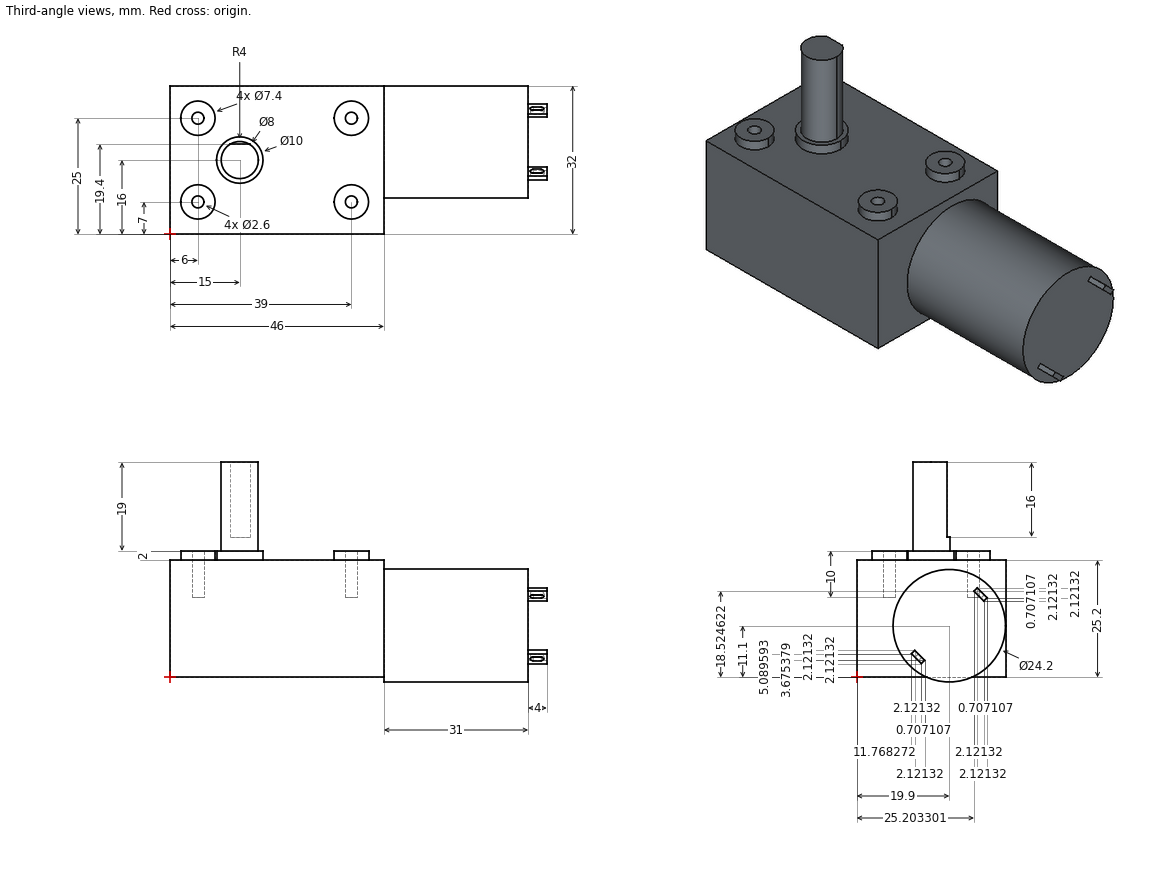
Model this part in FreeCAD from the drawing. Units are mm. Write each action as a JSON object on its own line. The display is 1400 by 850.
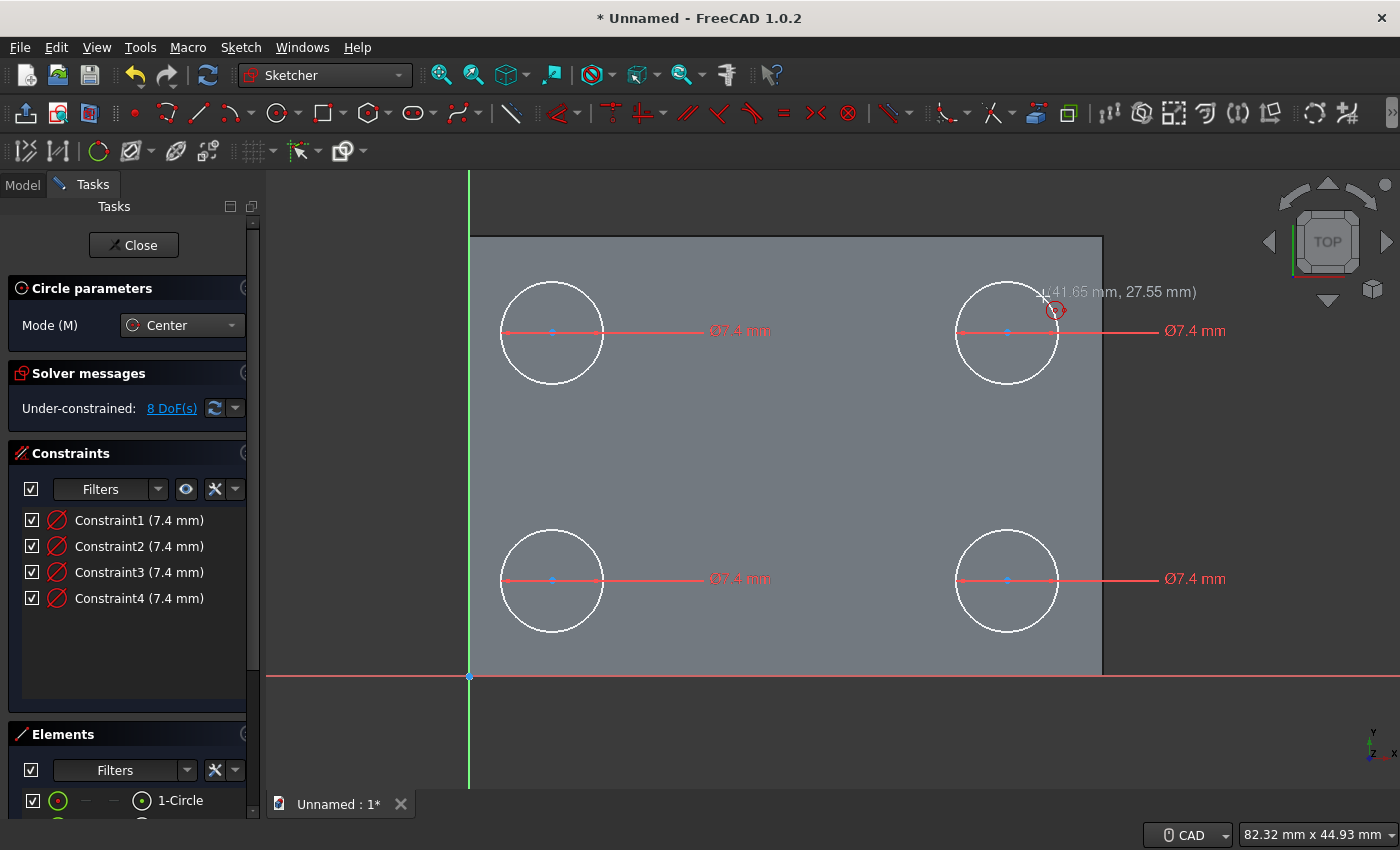
{"action": "left_click", "coordinate": [676, 456]}
{"action": "mouse_move", "coordinate": [725, 407]}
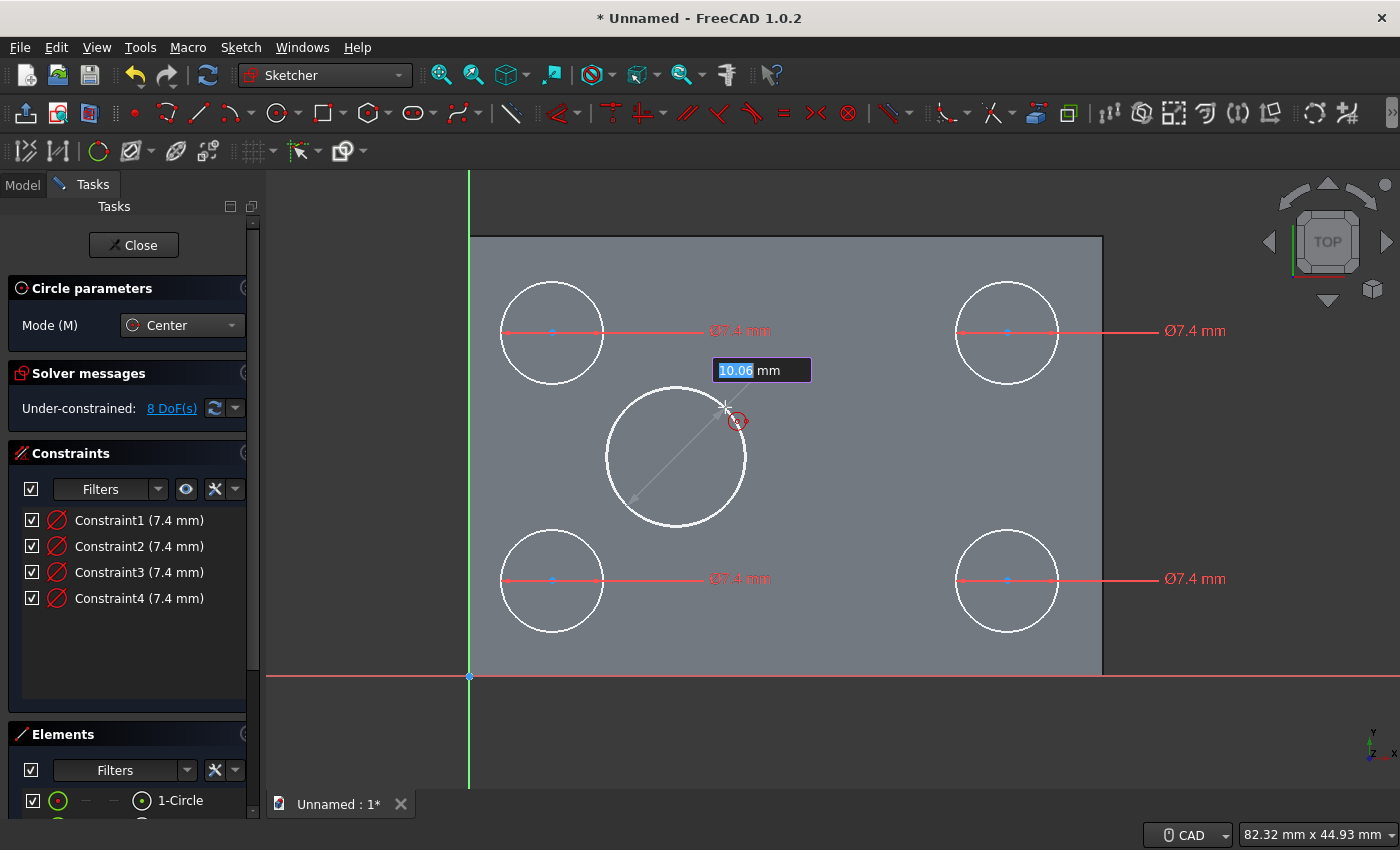
{"action": "type", "text": "10"}
{"action": "key", "text": "Return"}
{"action": "key", "text": "Escape"}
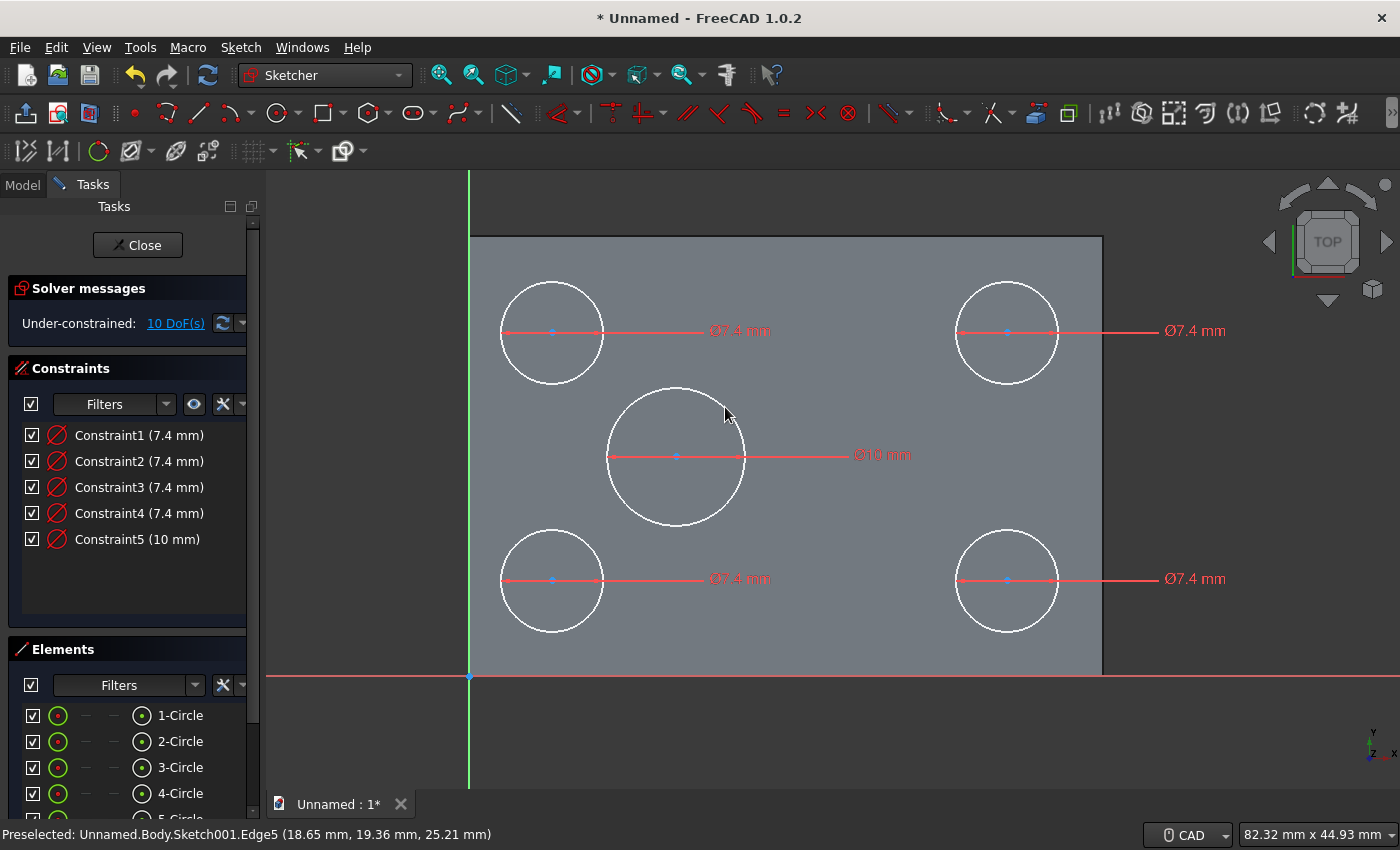
{"action": "left_click", "coordinate": [552, 333]}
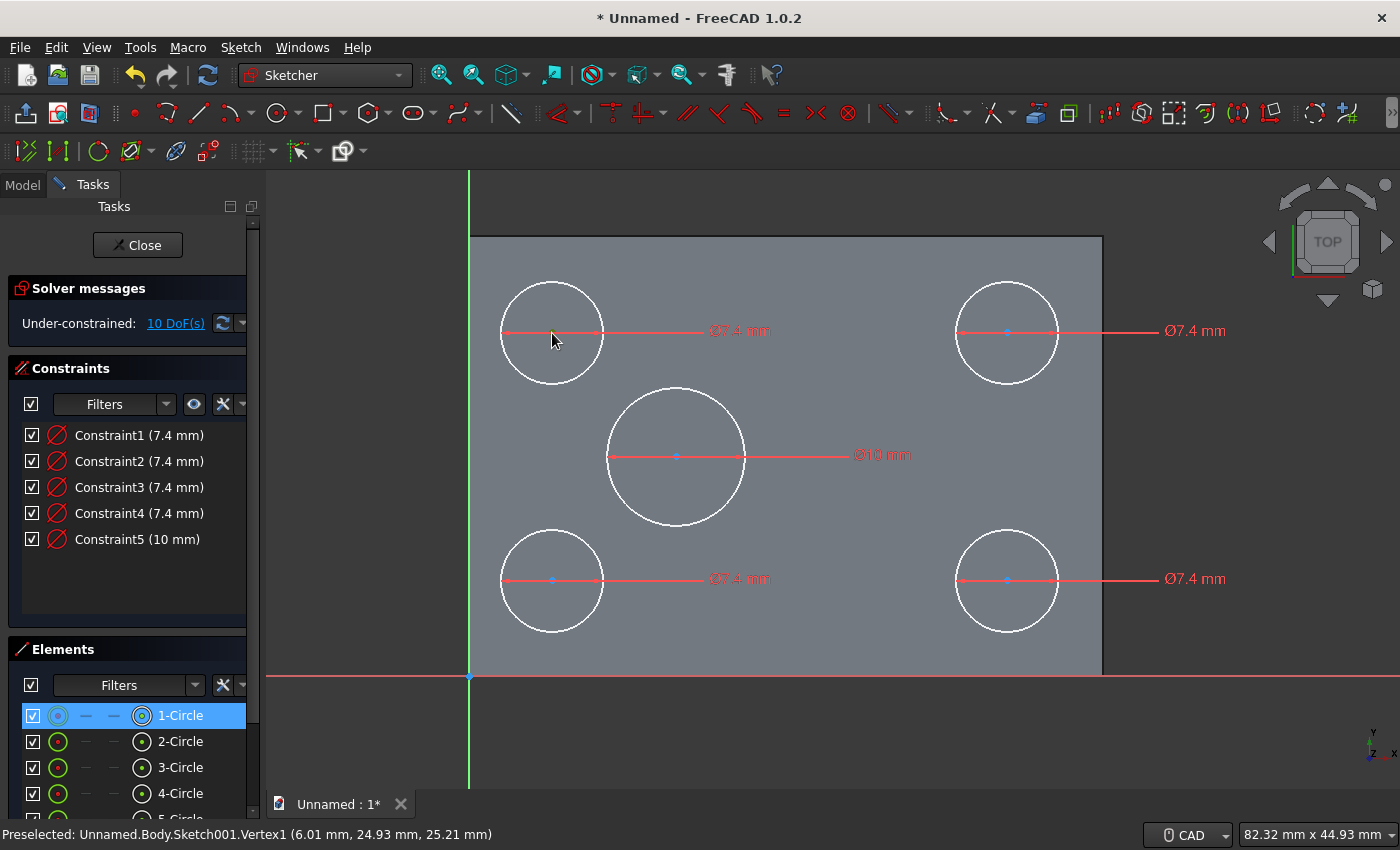
{"action": "left_click", "coordinate": [552, 581]}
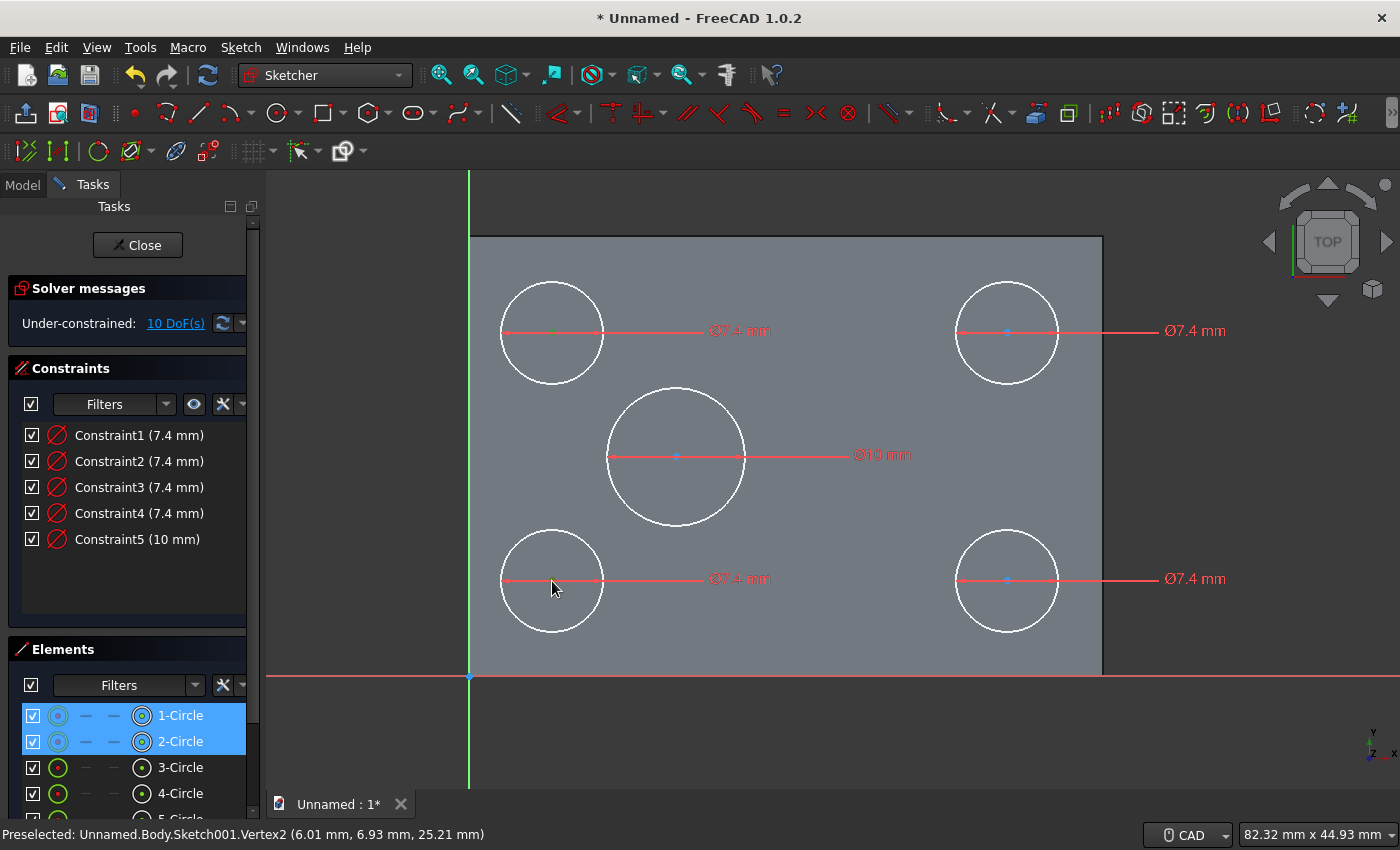
{"action": "left_click", "coordinate": [666, 114]}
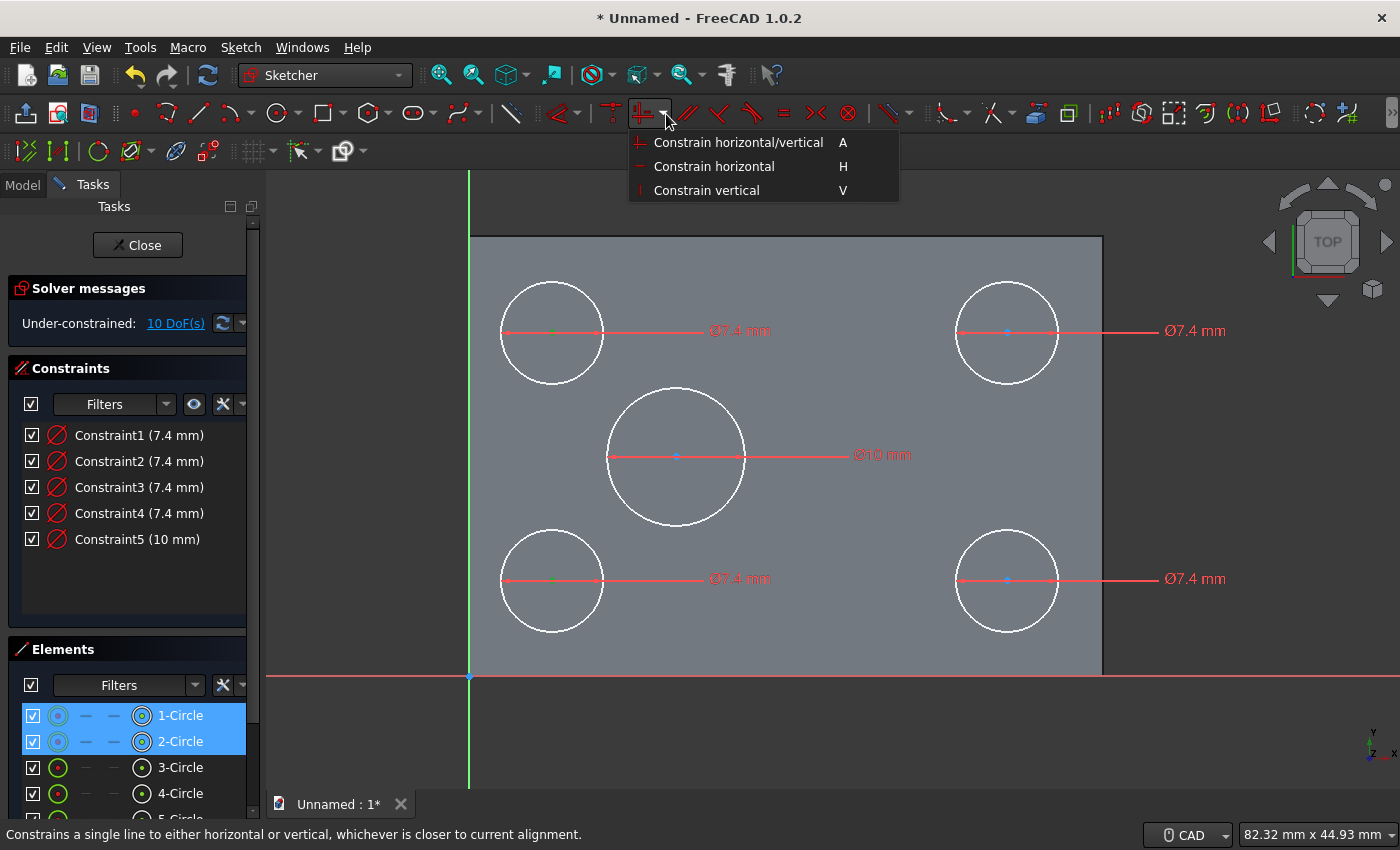
{"action": "left_click", "coordinate": [764, 190]}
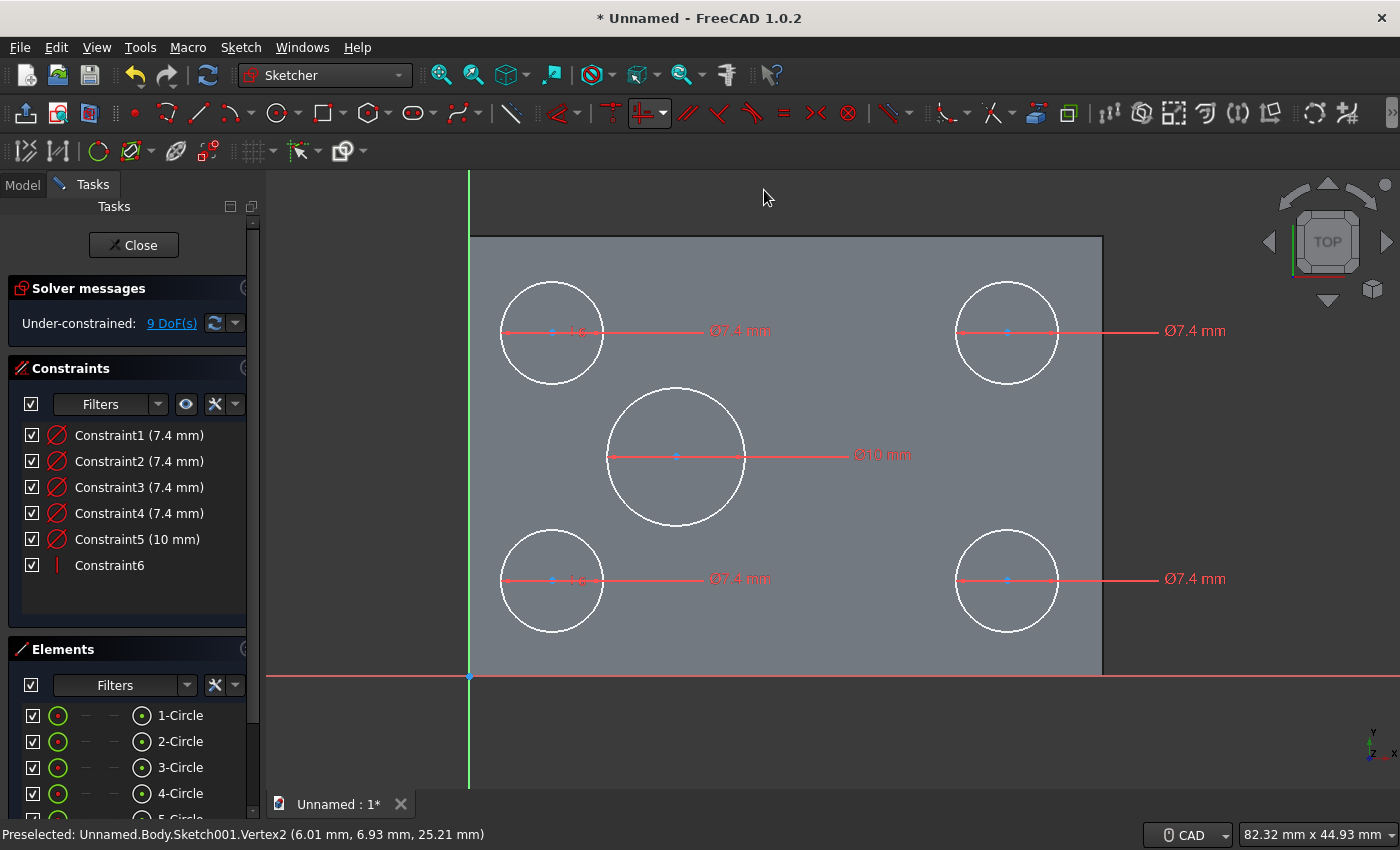
{"action": "left_click", "coordinate": [552, 581]}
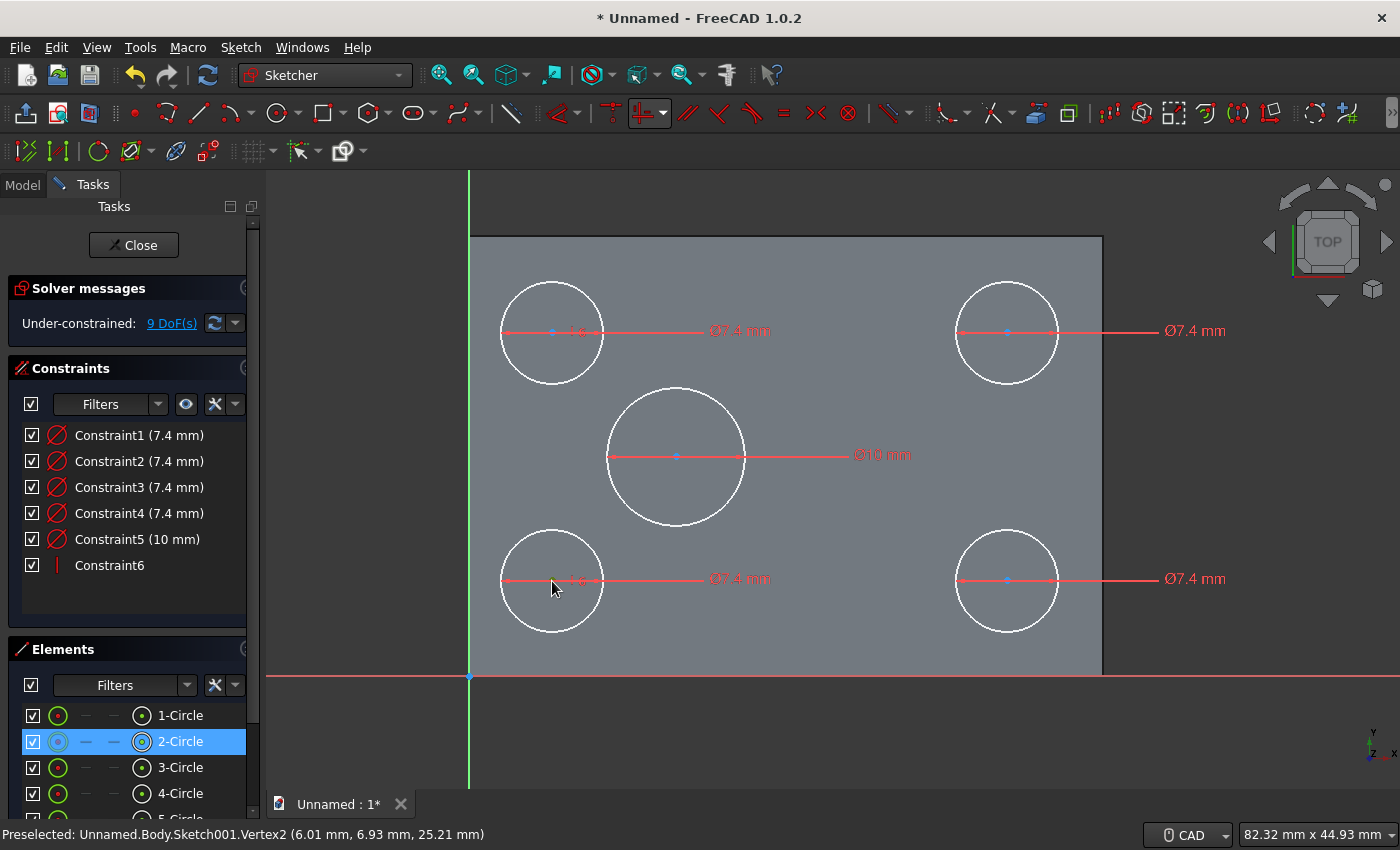
{"action": "left_click", "coordinate": [1007, 581]}